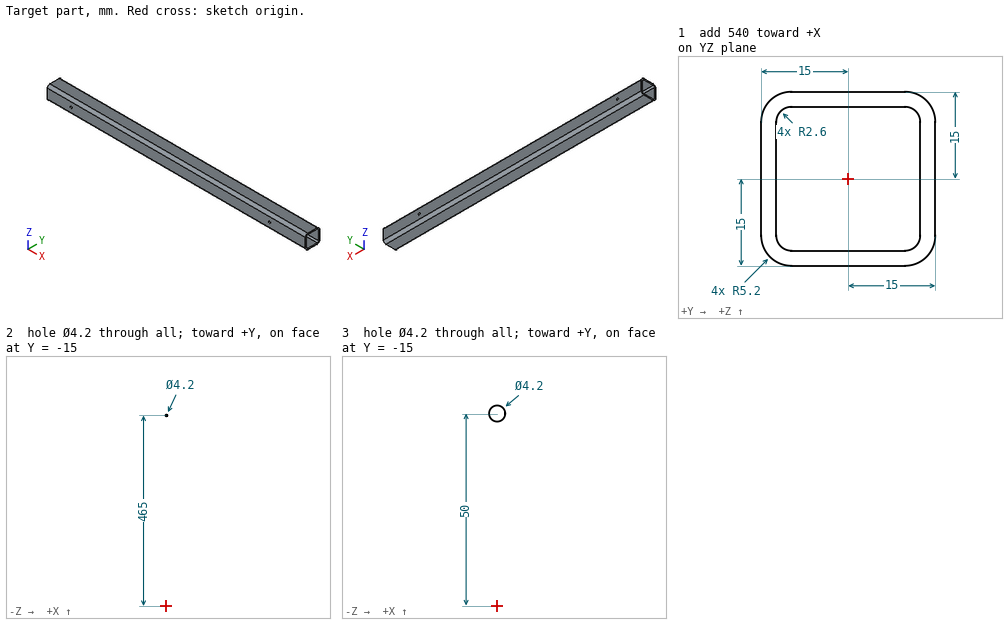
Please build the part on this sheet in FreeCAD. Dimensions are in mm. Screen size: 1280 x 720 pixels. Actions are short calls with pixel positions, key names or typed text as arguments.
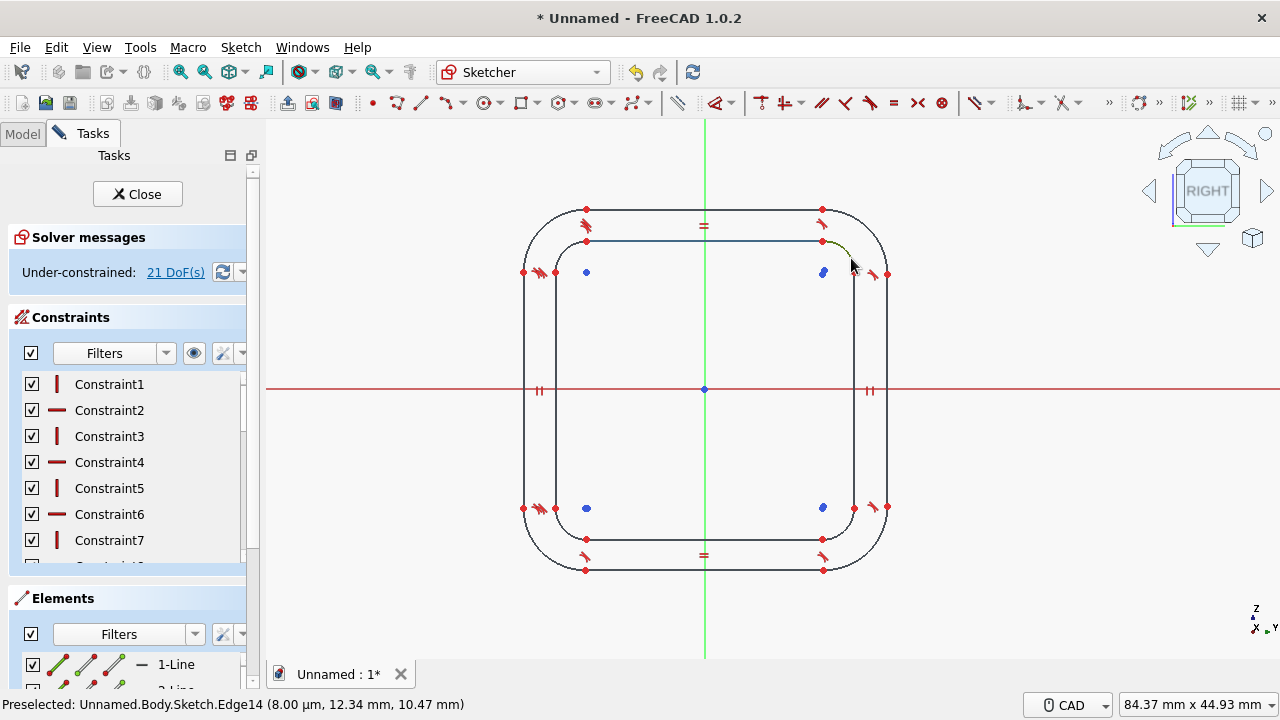
click(870, 104)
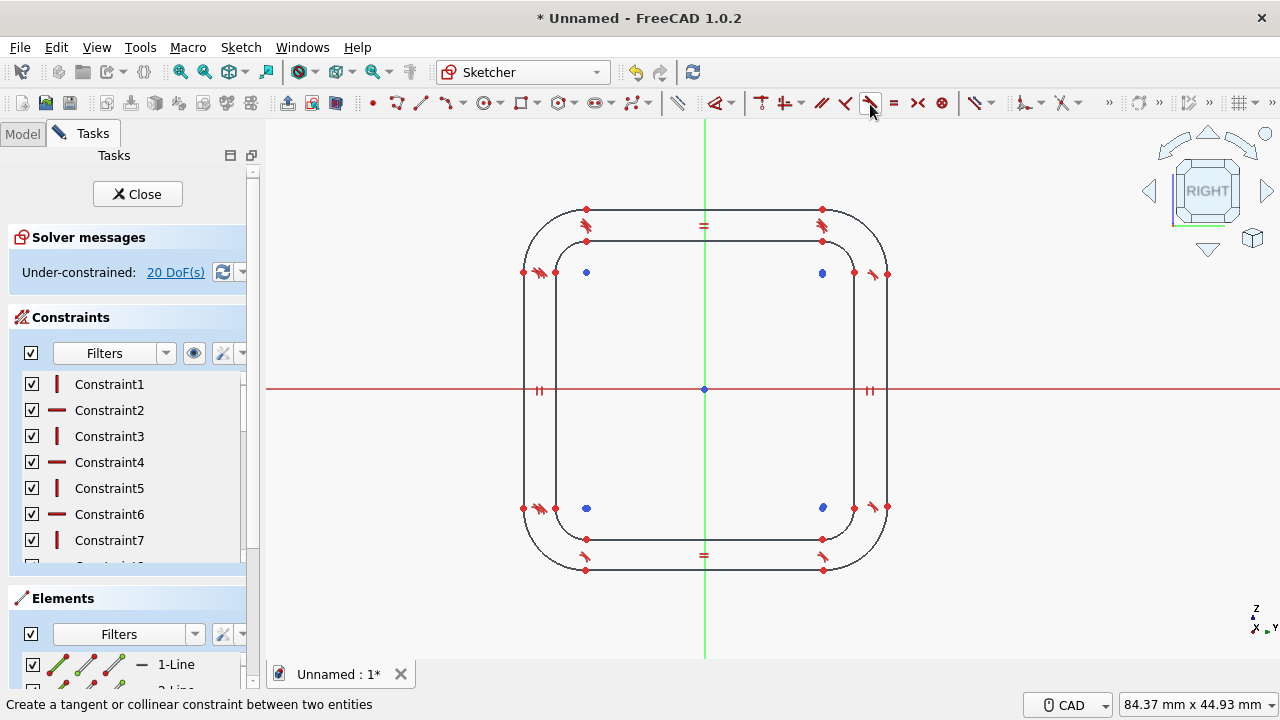
click(854, 343)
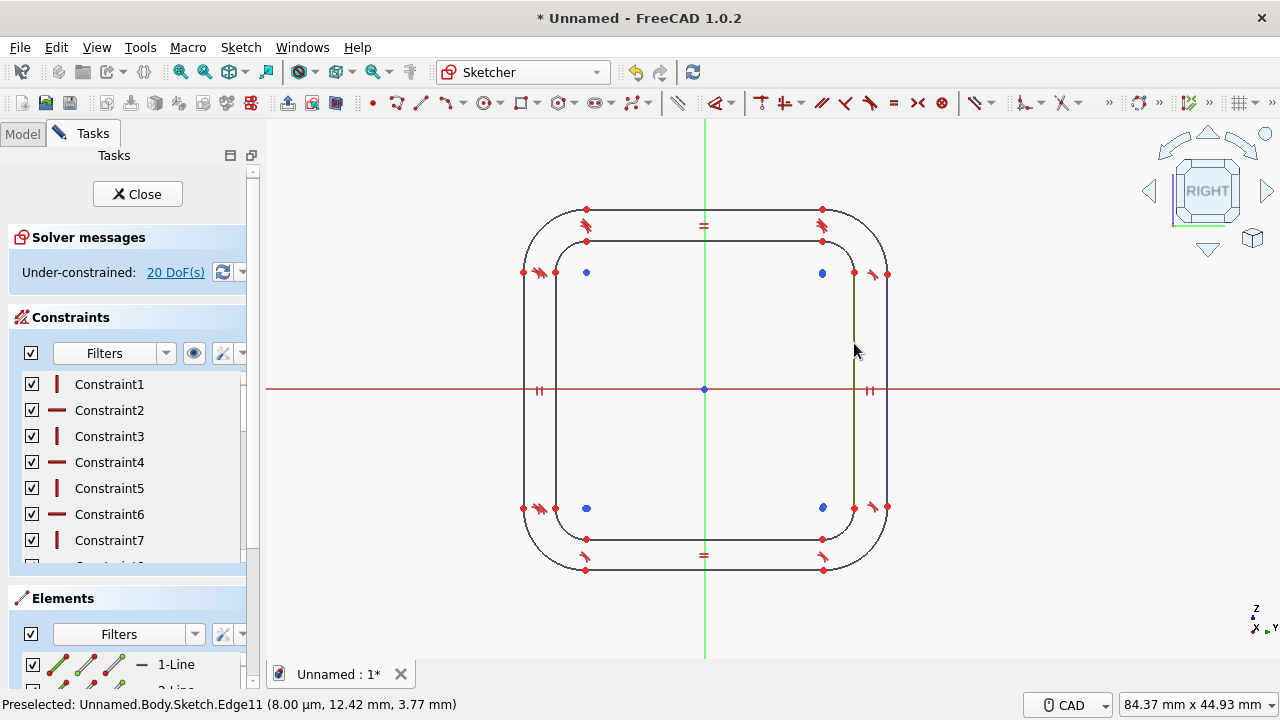
click(851, 258)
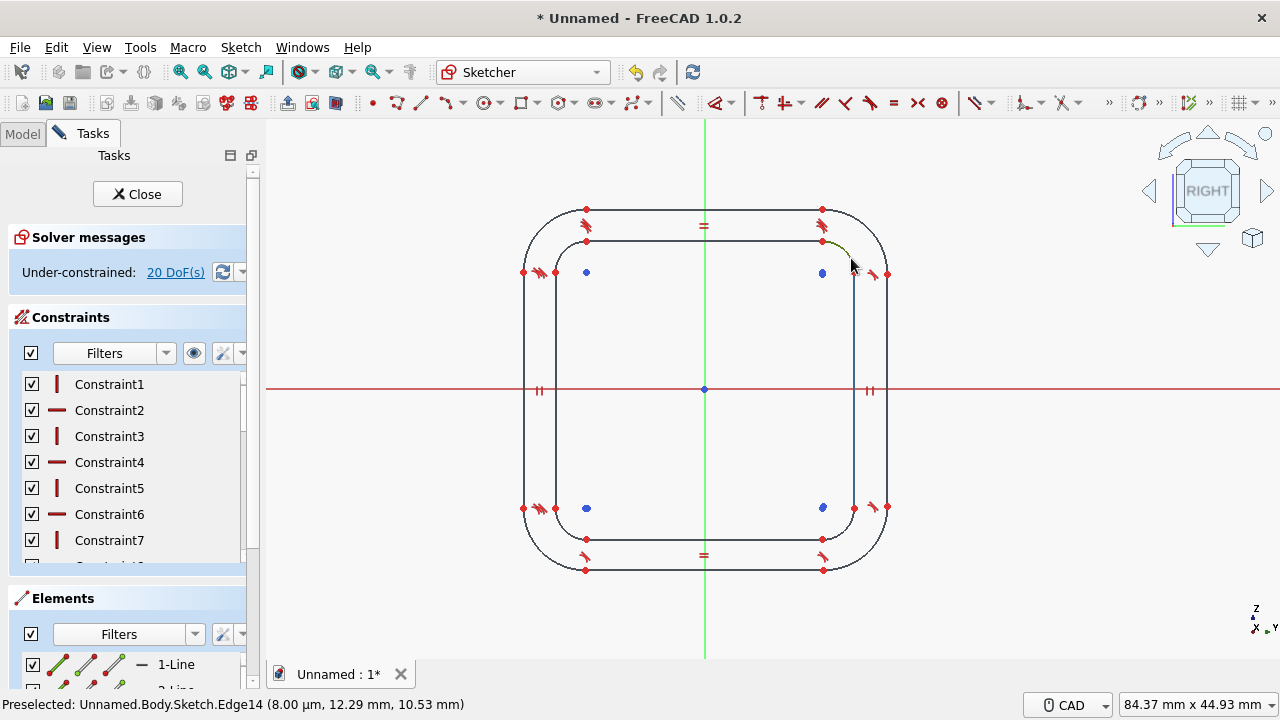
click(870, 104)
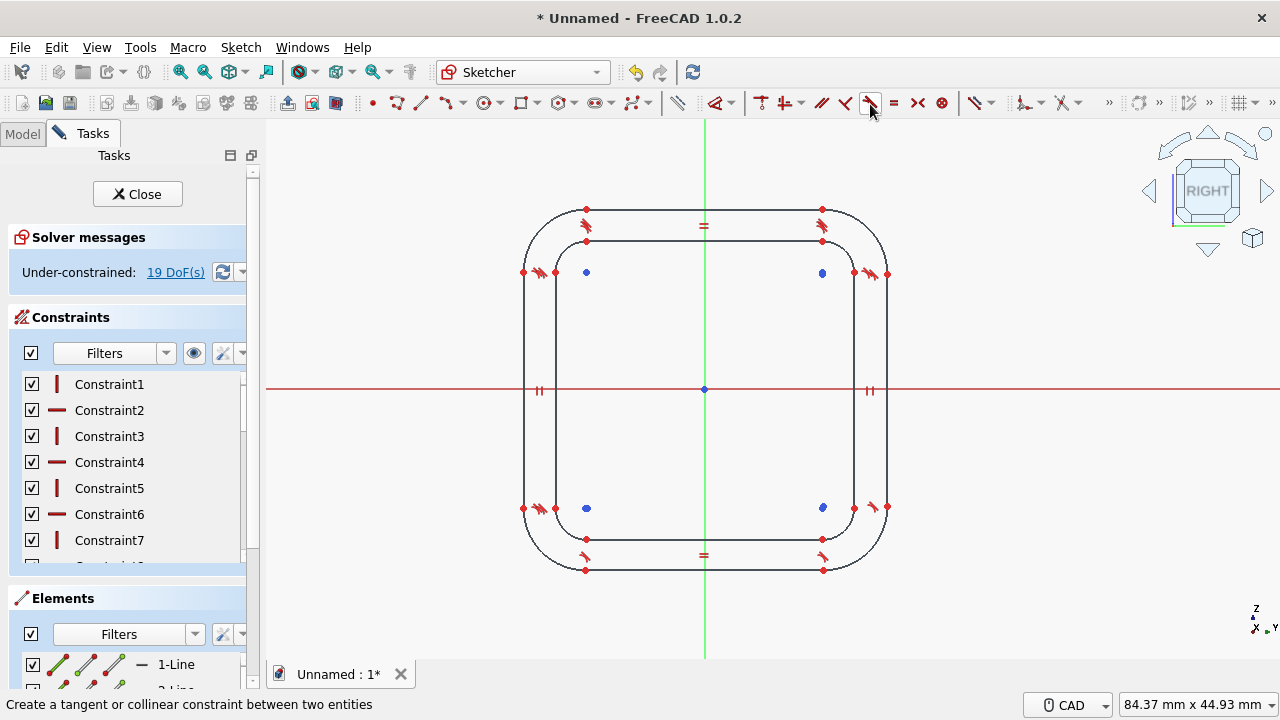
click(854, 343)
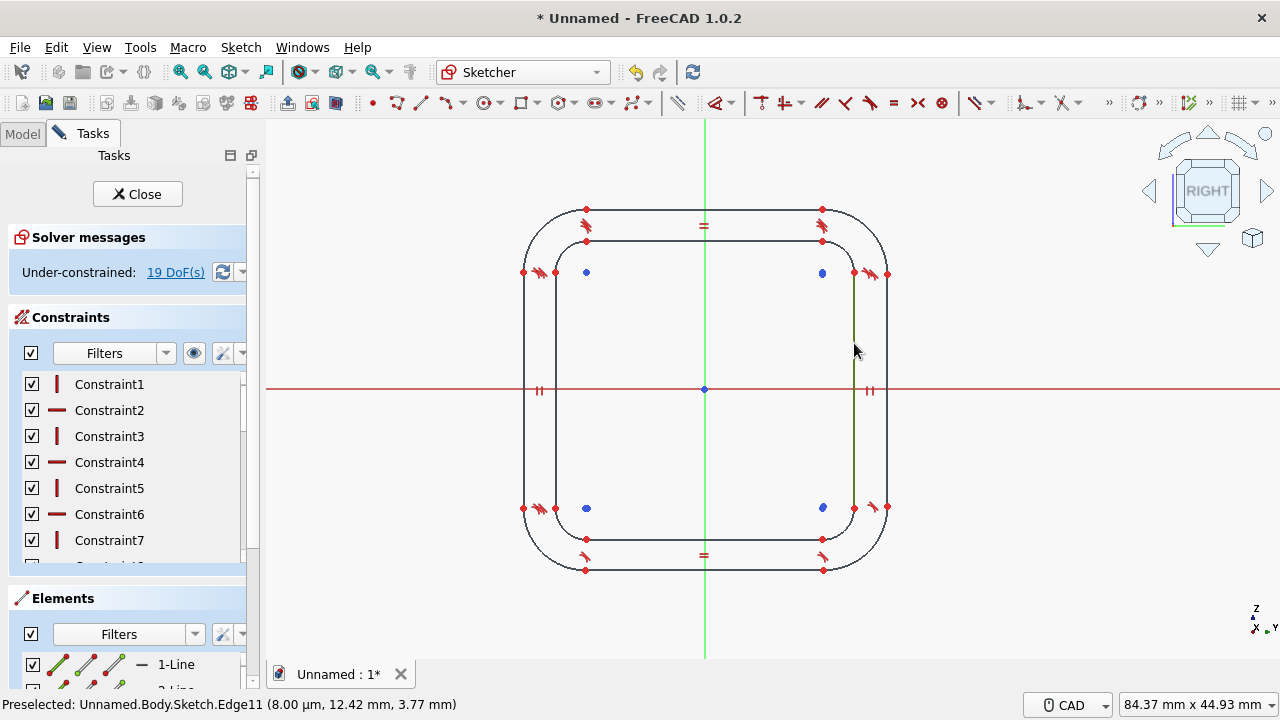
click(837, 536)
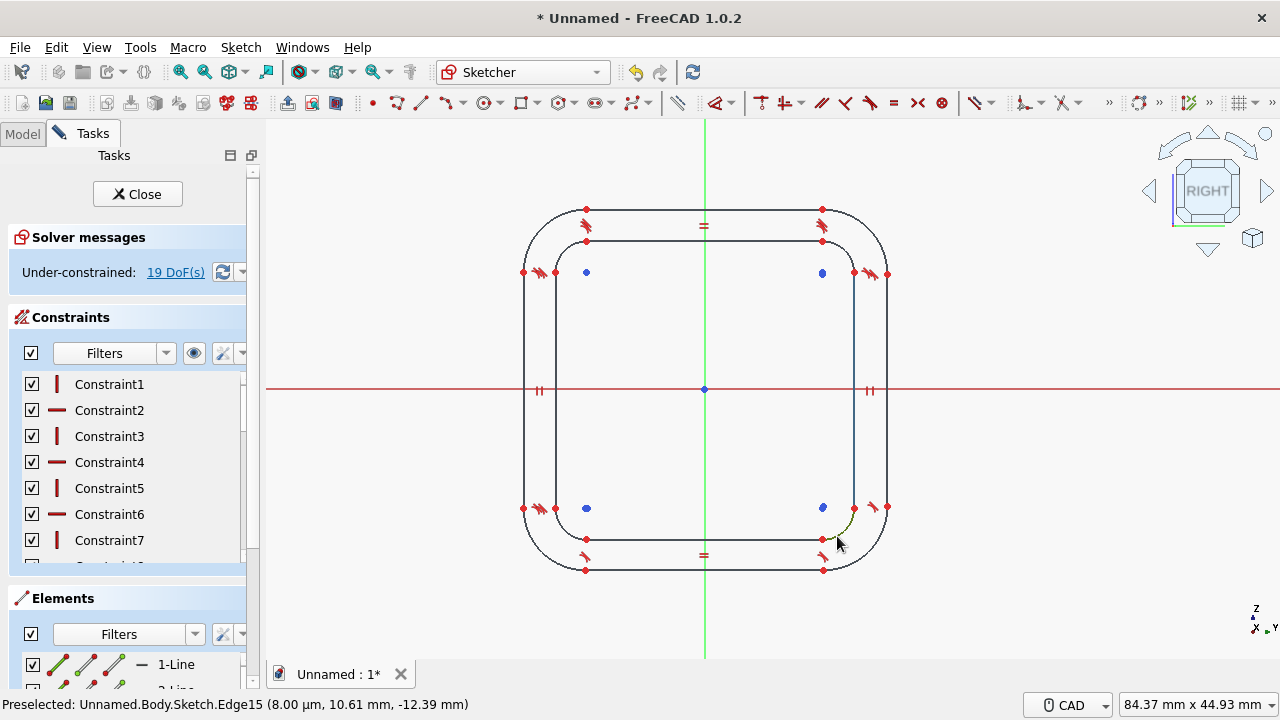
click(870, 104)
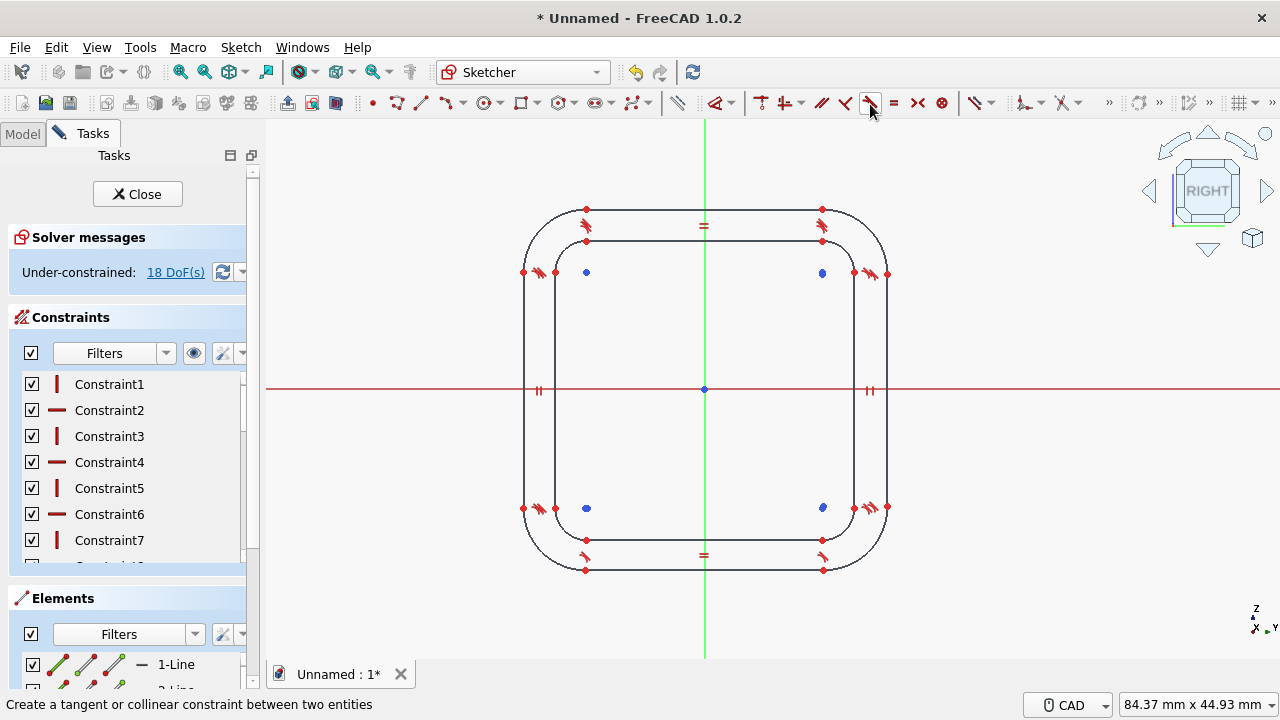
click(752, 540)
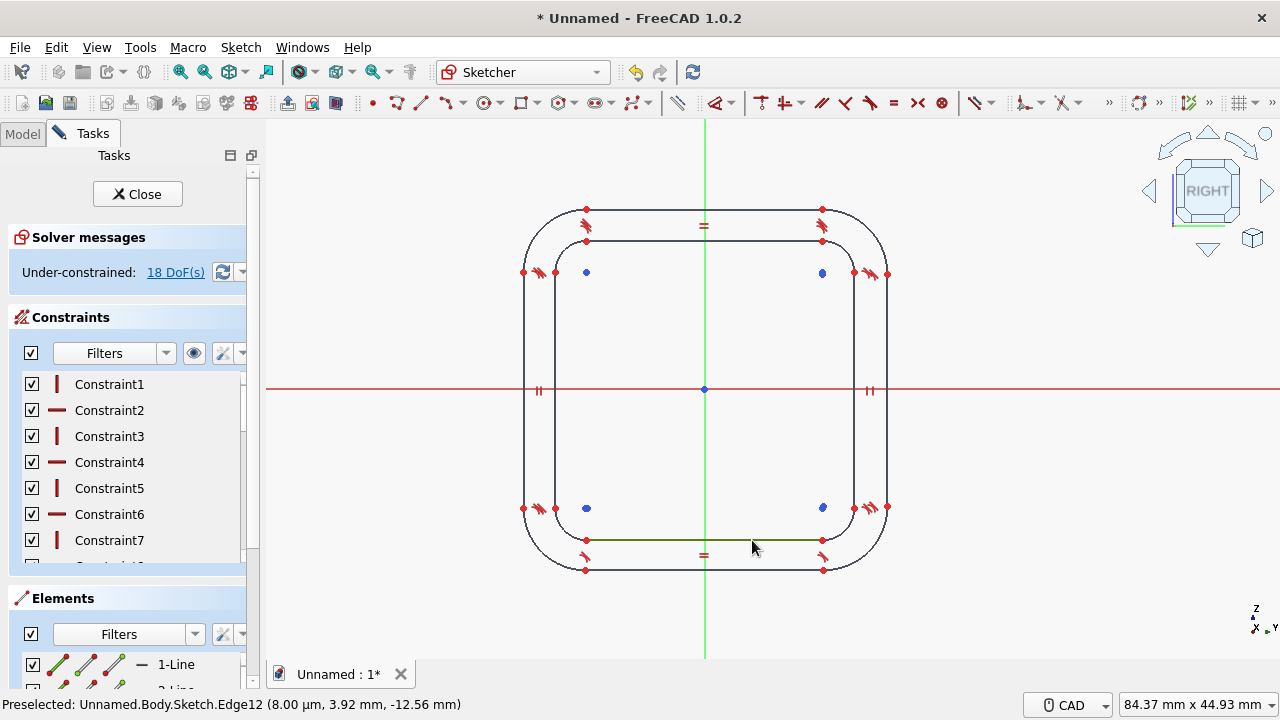
click(837, 537)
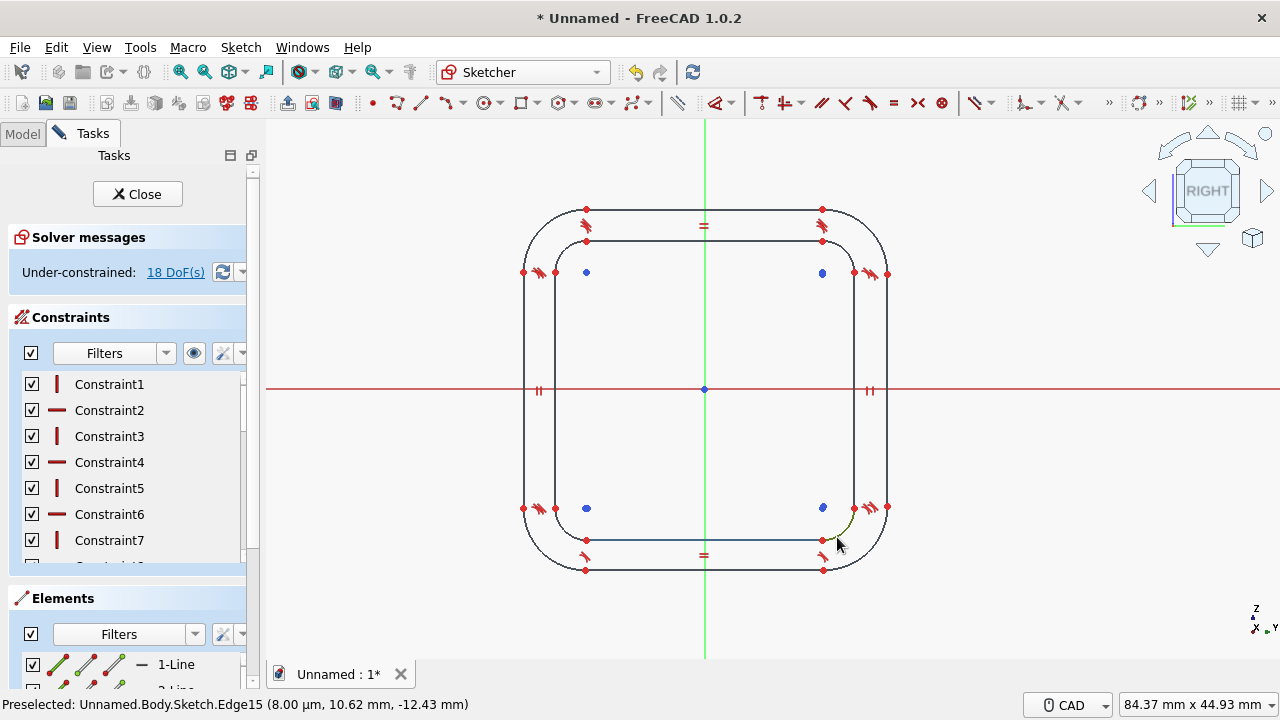
click(870, 104)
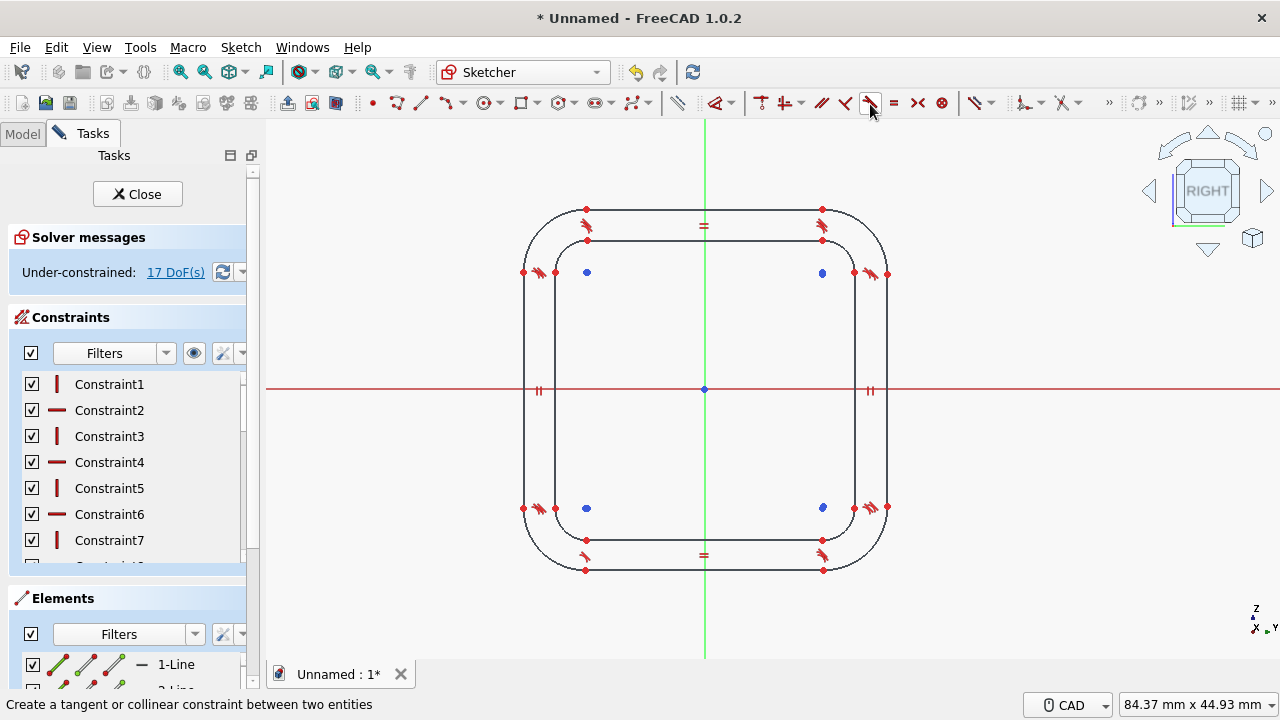
click(752, 540)